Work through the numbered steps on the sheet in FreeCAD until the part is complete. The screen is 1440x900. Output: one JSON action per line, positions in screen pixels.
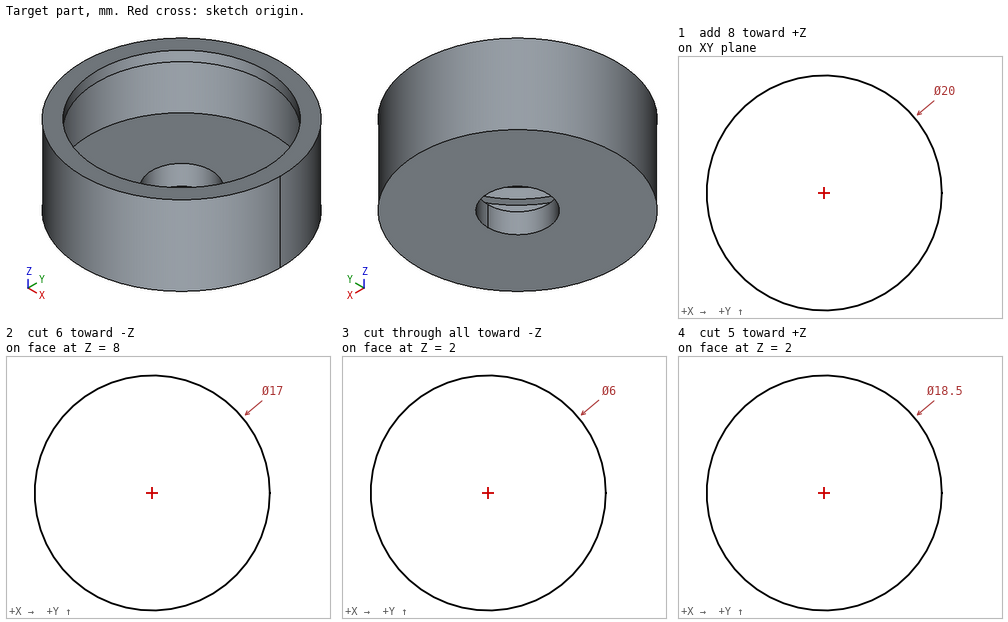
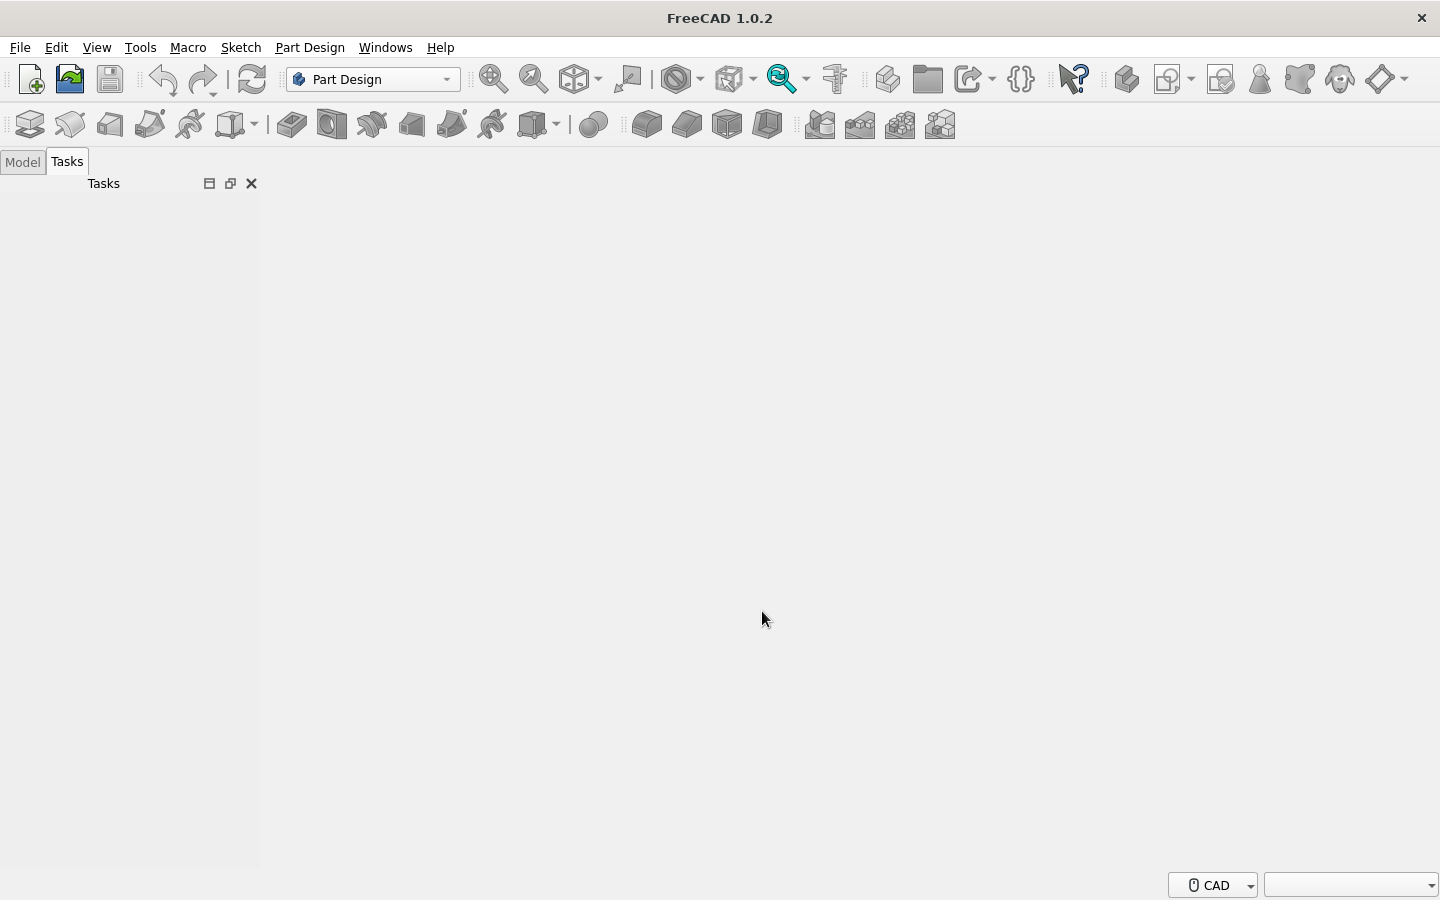
{"action": "key", "text": "ctrl+n"}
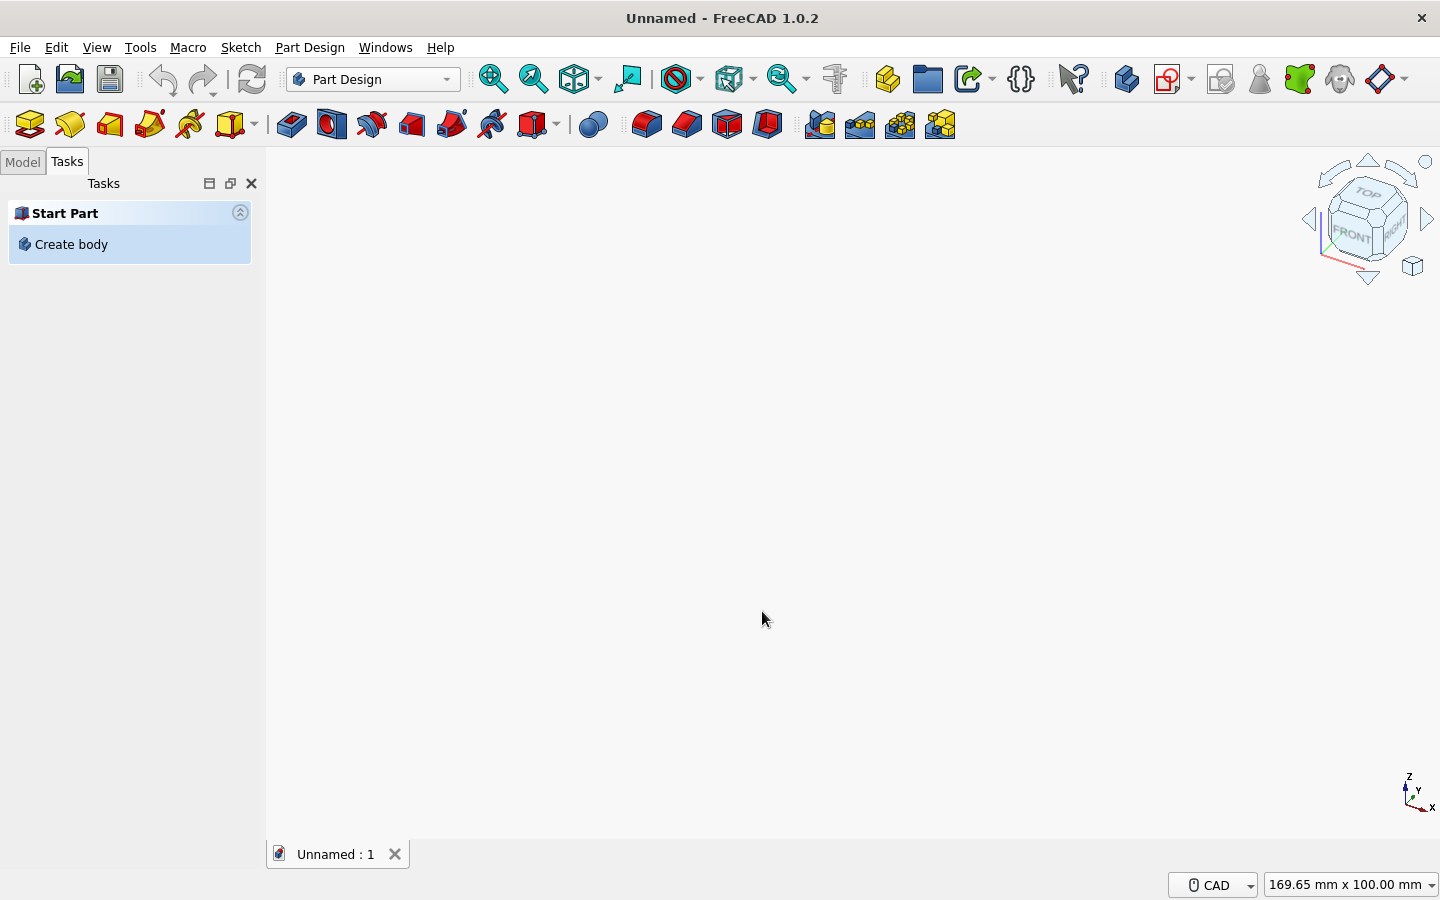
{"action": "left_click", "coordinate": [1168, 80]}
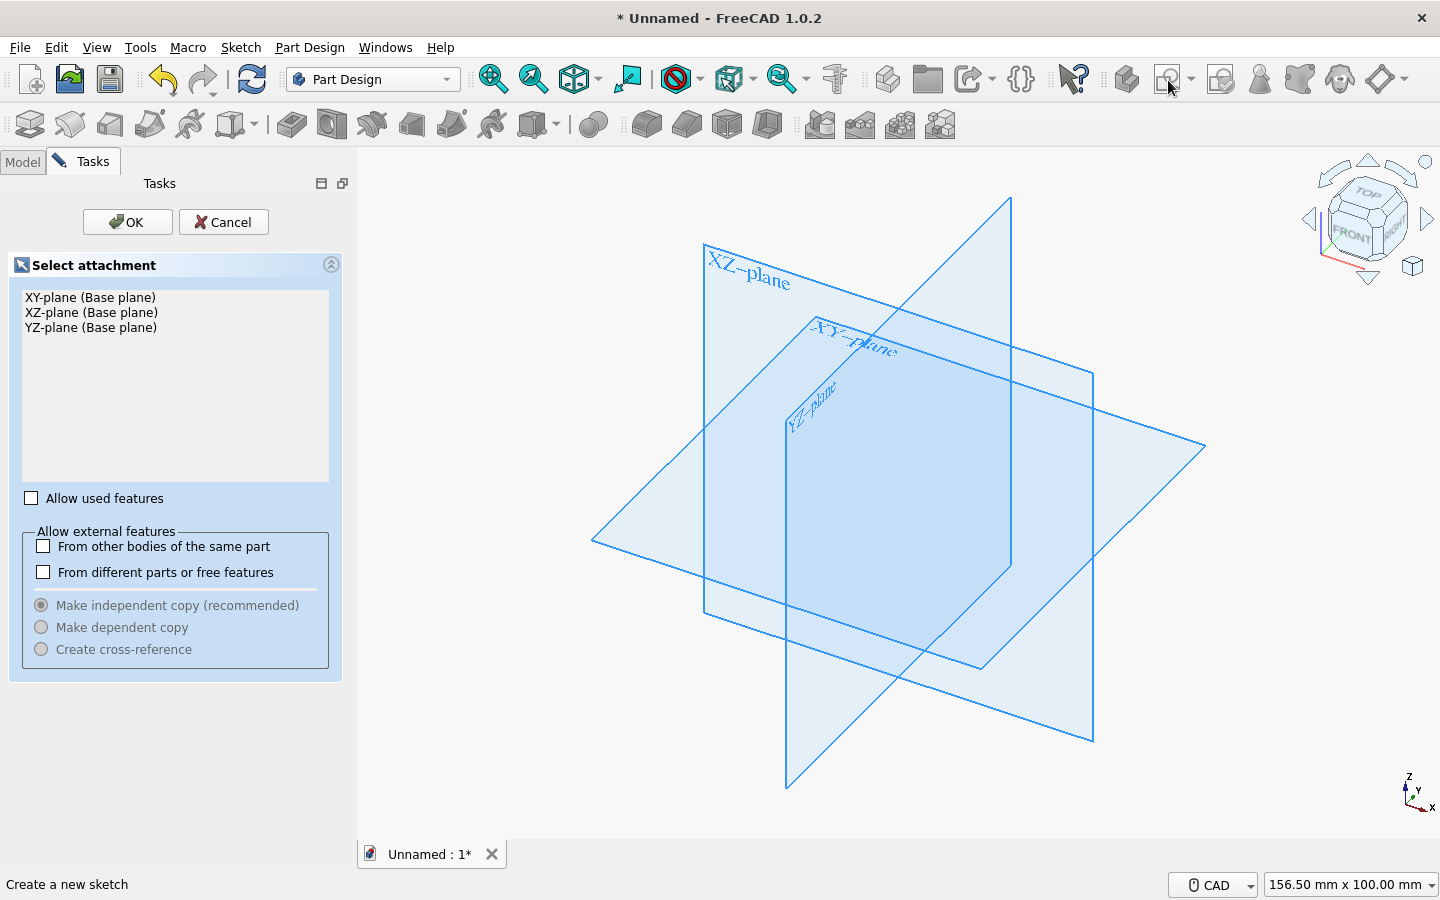
{"action": "left_click", "coordinate": [82, 298]}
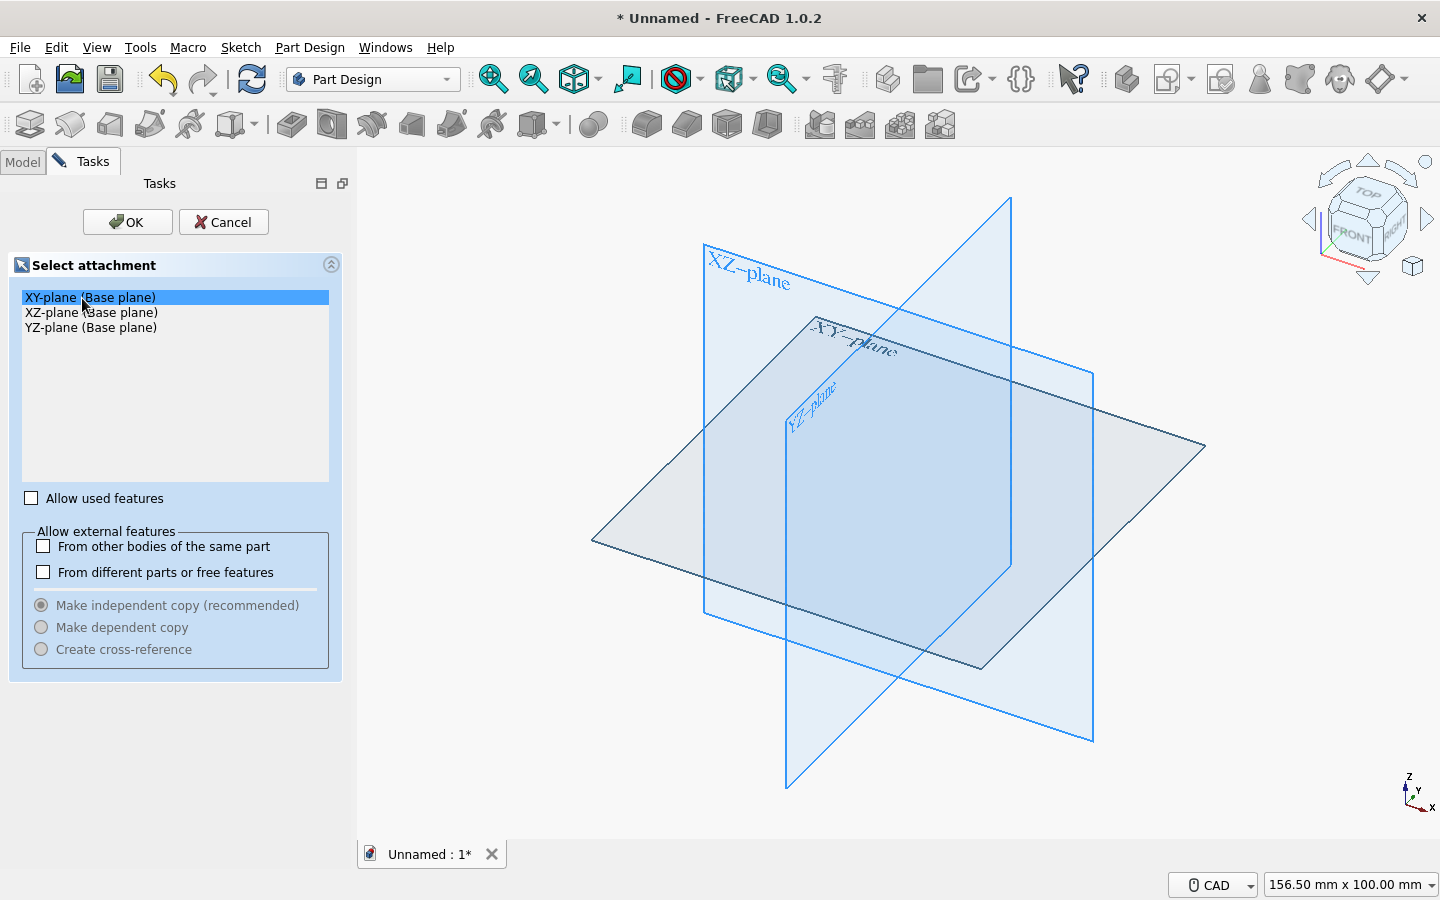
{"action": "left_click", "coordinate": [128, 222]}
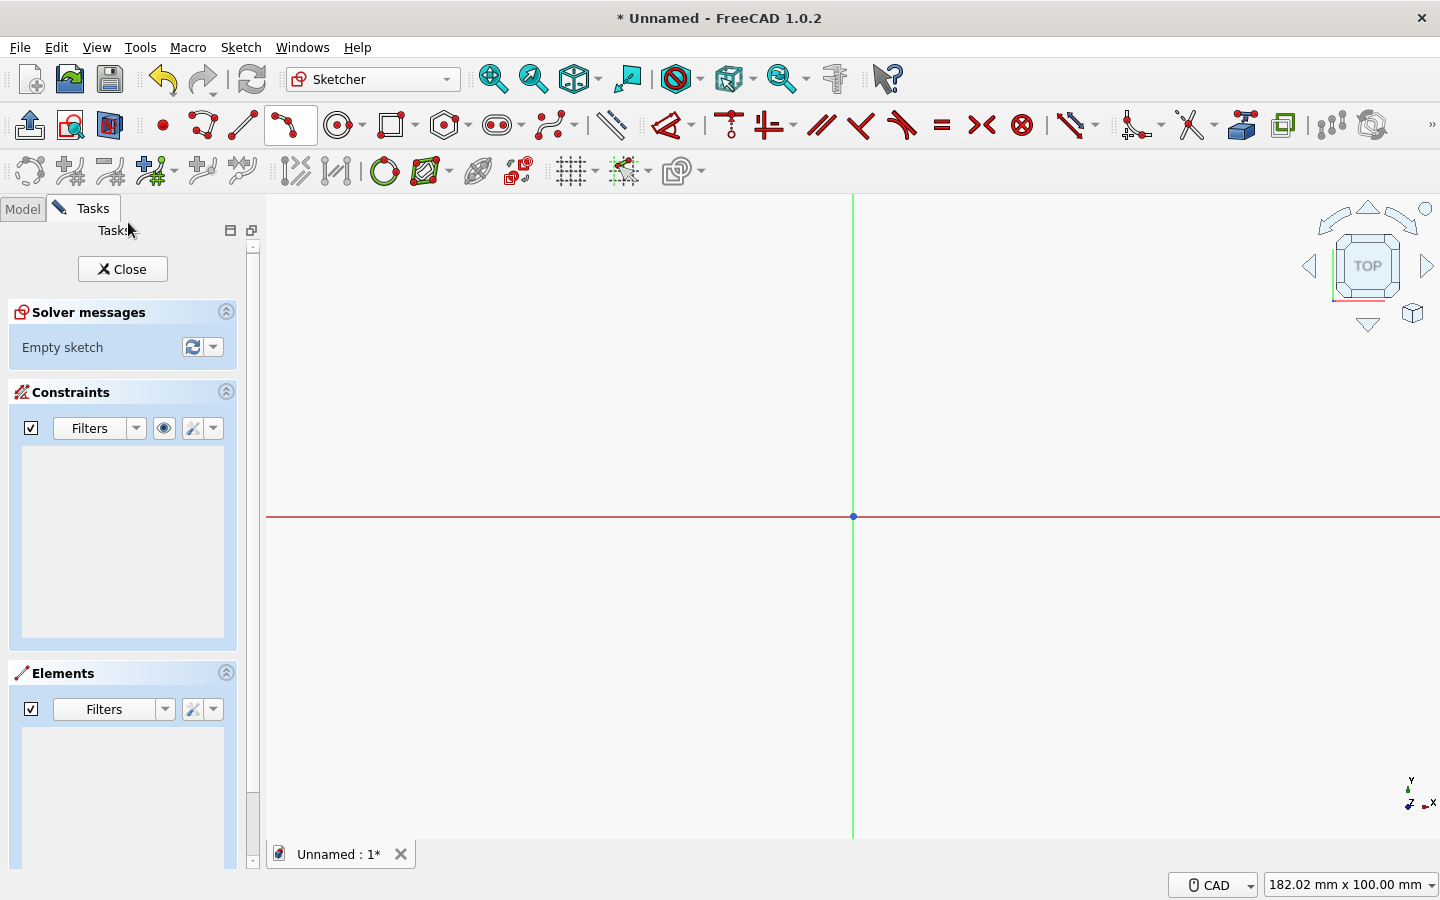
{"action": "scroll", "coordinate": [883, 516], "scroll_direction": "up", "scroll_amount": 6}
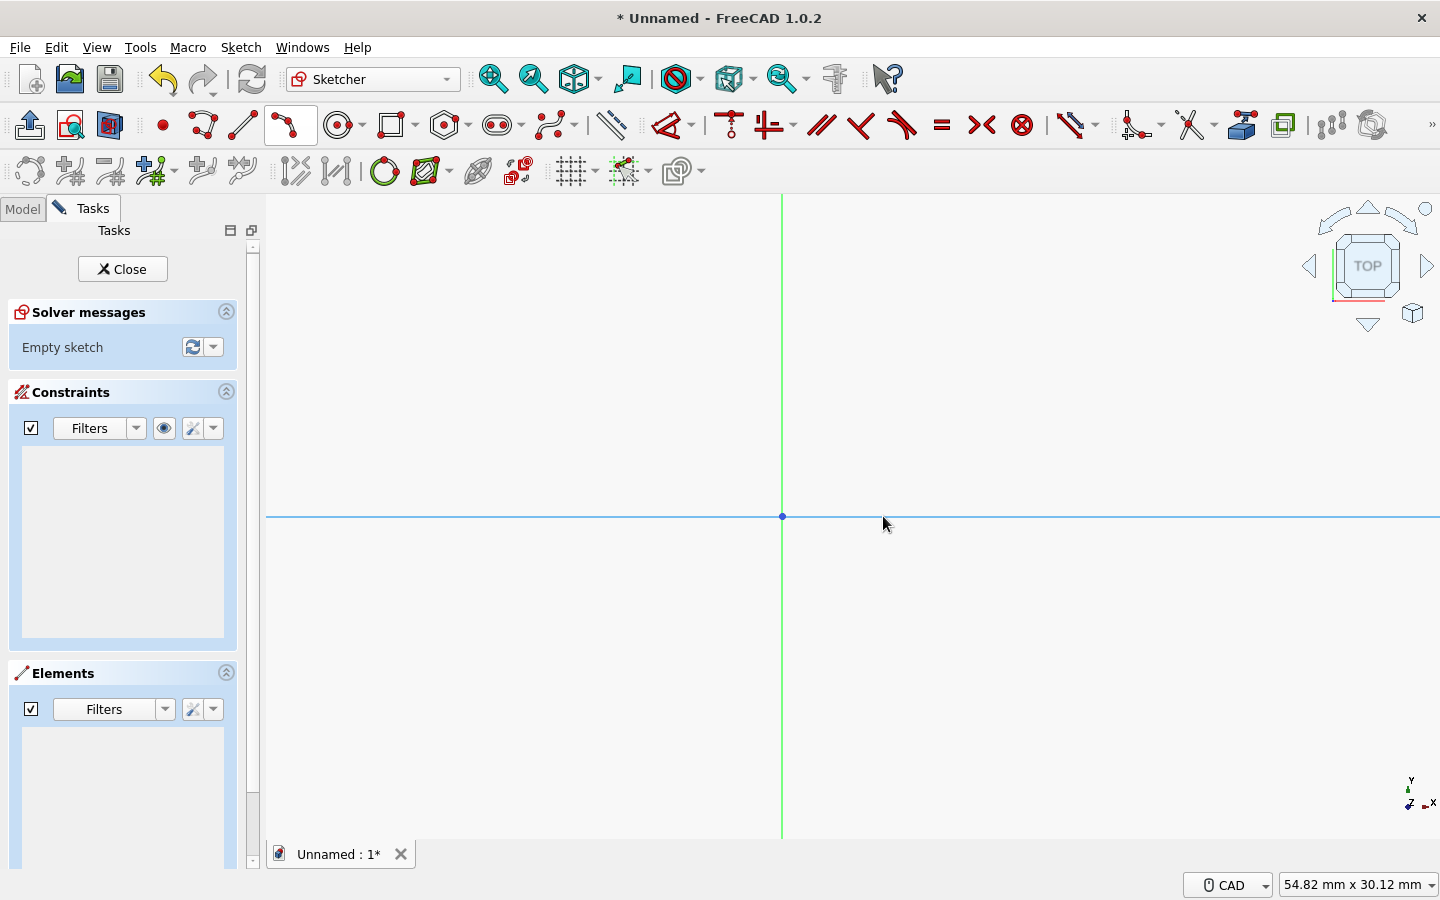
{"action": "left_click", "coordinate": [338, 126]}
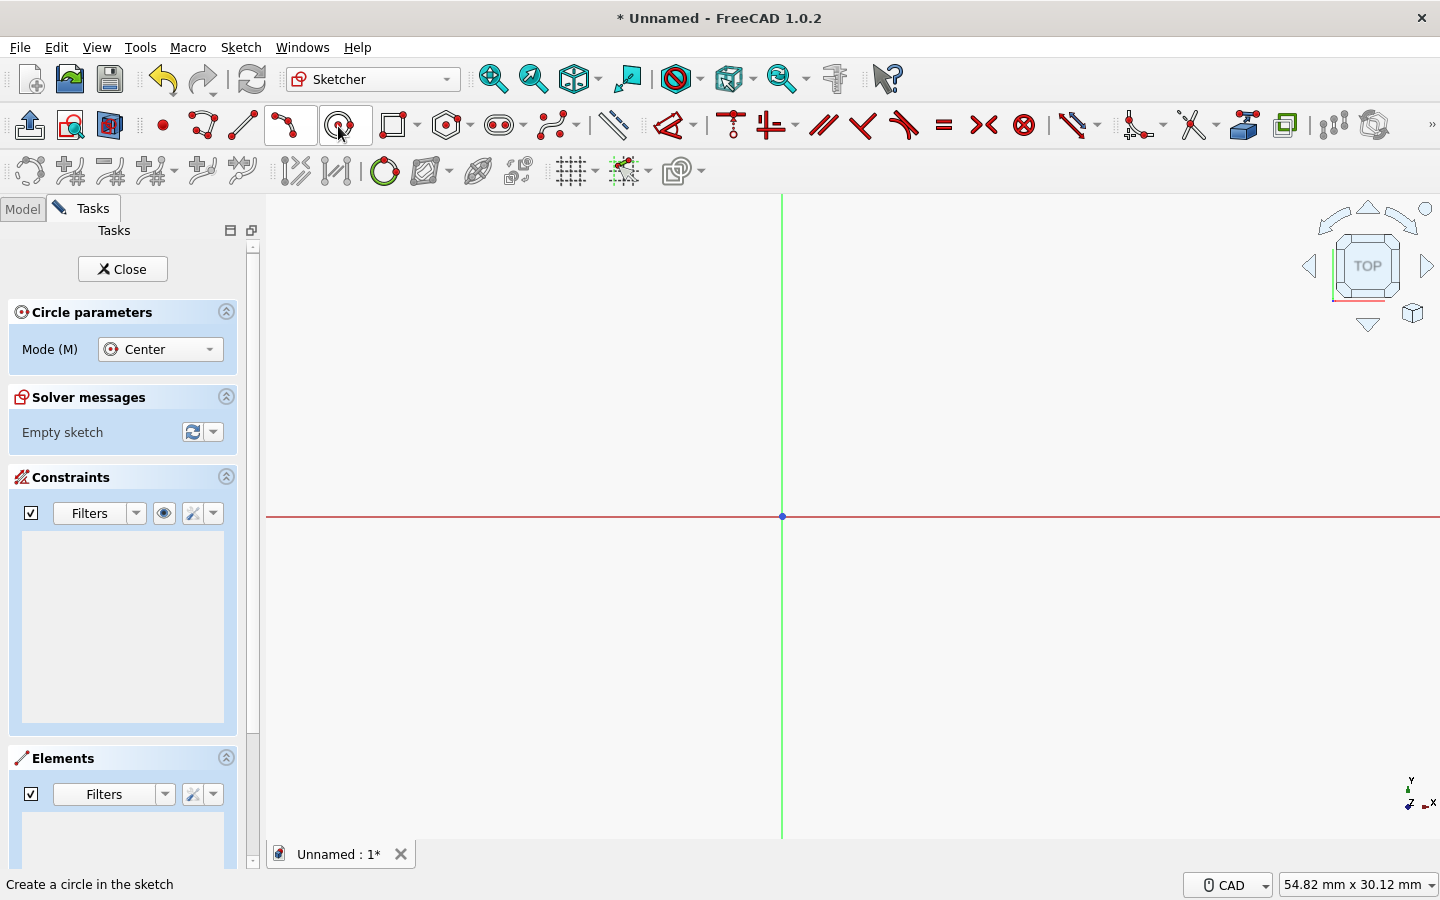
{"action": "left_click", "coordinate": [782, 516]}
{"action": "mouse_move", "coordinate": [934, 365]}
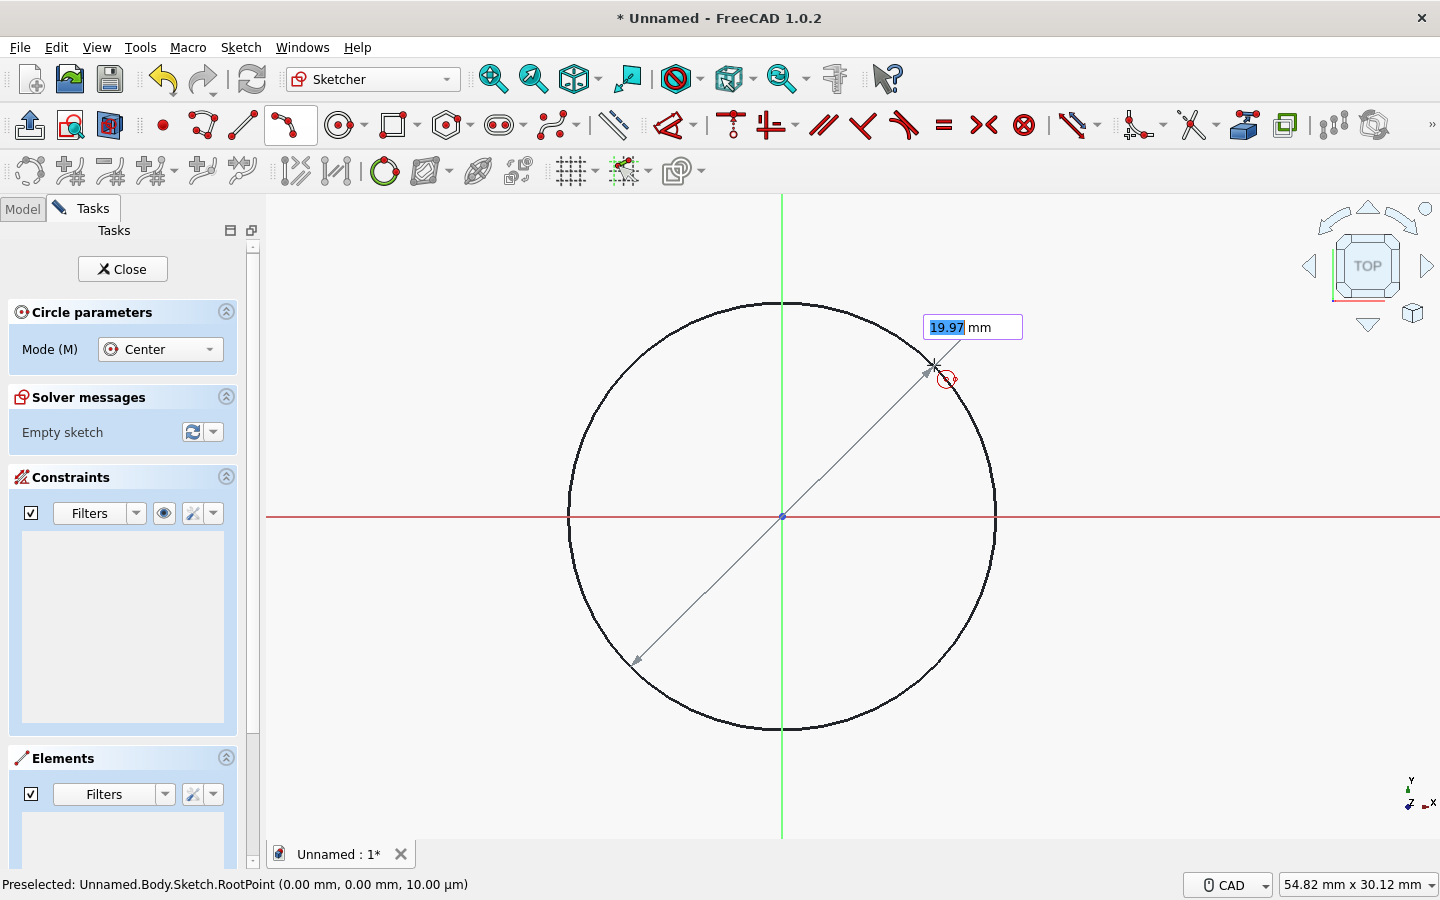
{"action": "type", "text": "20"}
{"action": "key", "text": "Return"}
{"action": "key", "text": "Escape"}